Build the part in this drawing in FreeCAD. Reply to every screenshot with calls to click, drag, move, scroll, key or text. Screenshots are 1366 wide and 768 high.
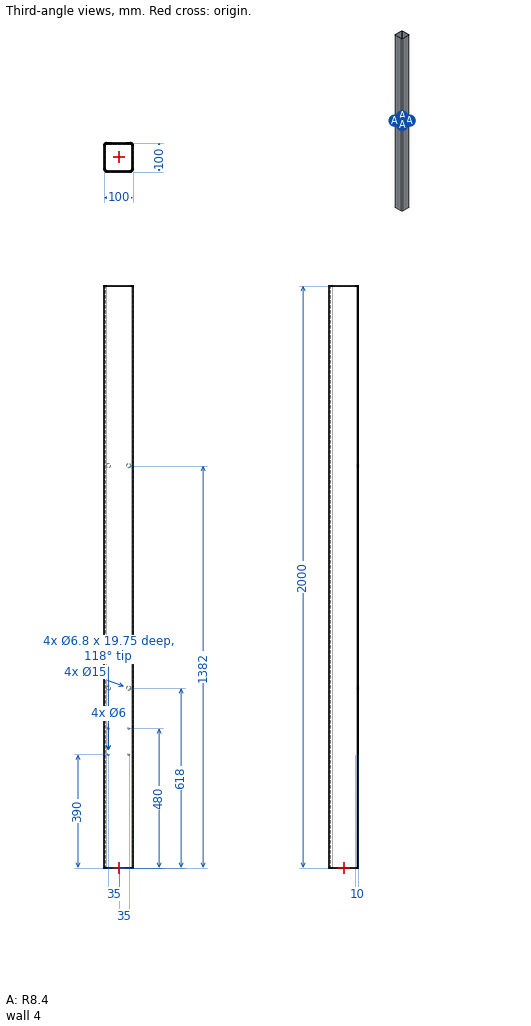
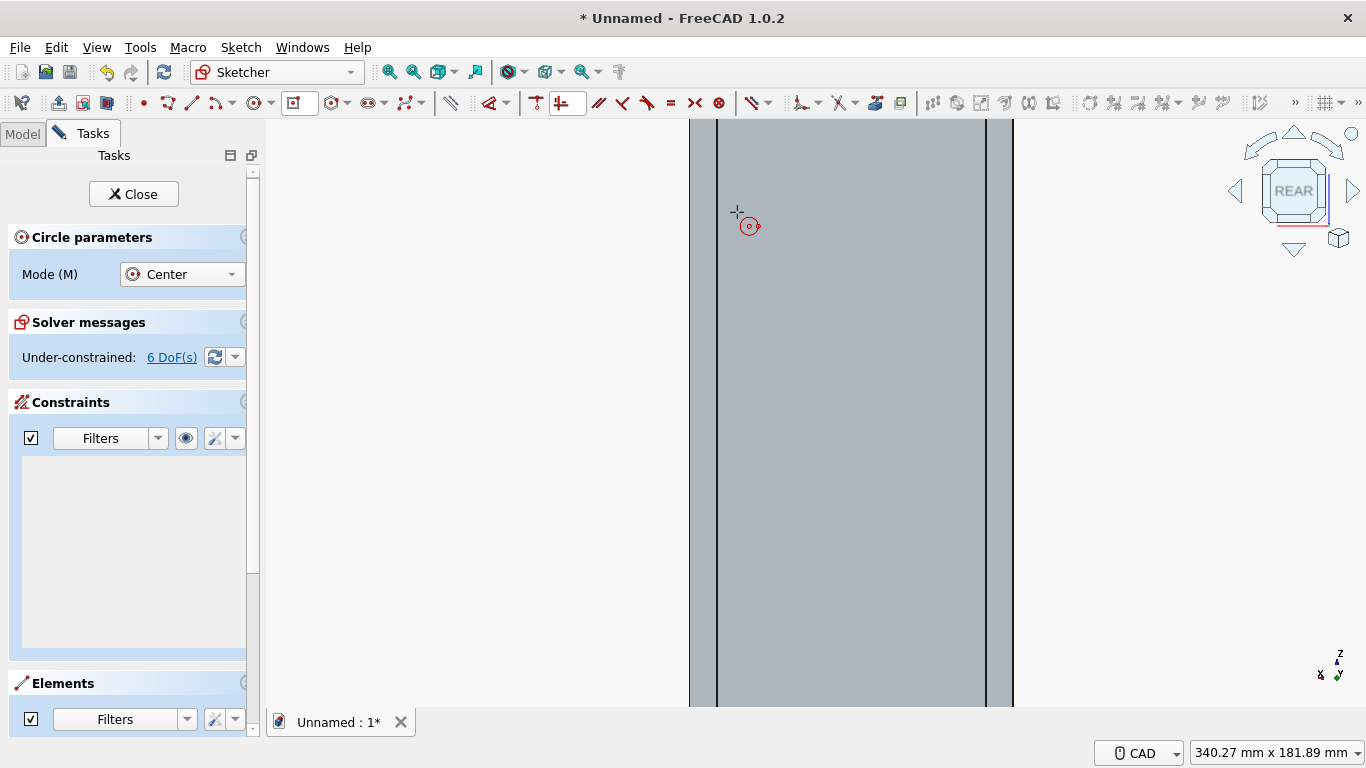
scroll(737, 212, down, 12)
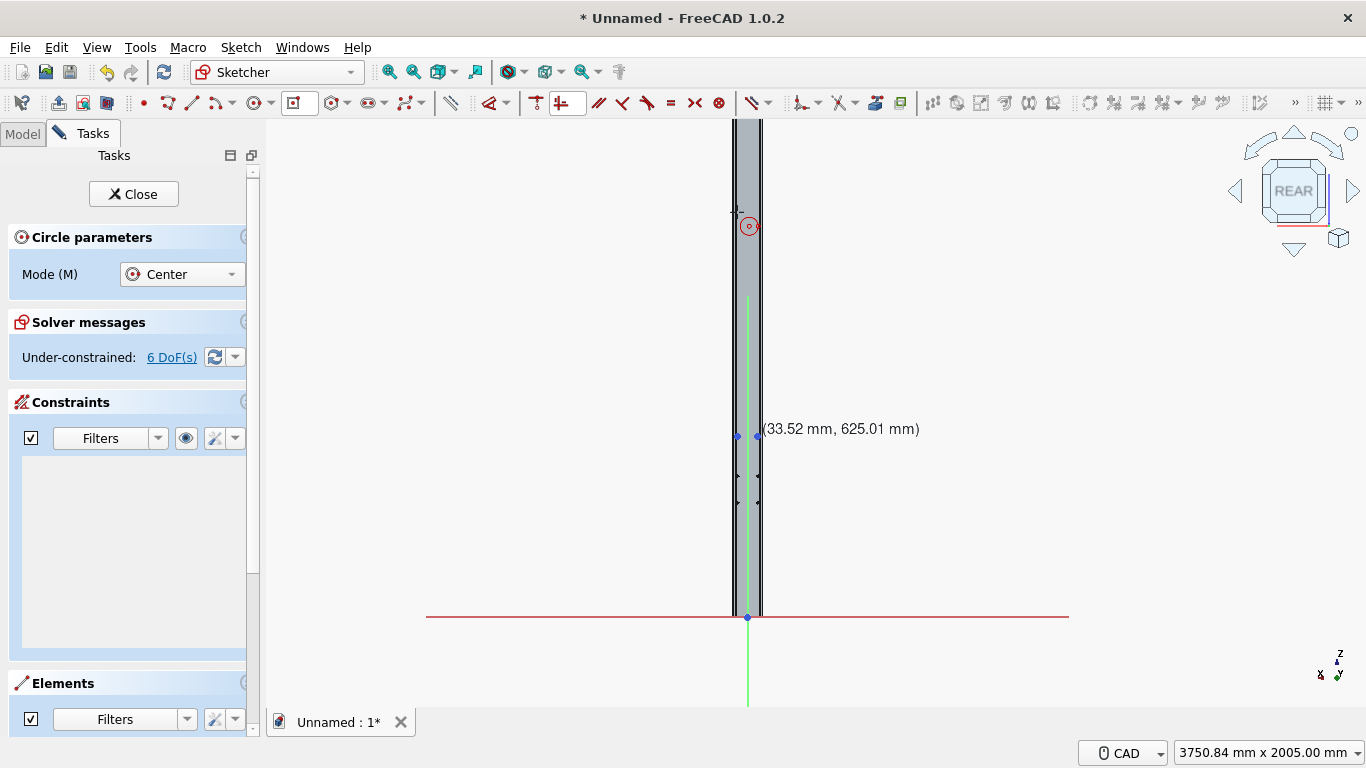
scroll(737, 212, up, 3)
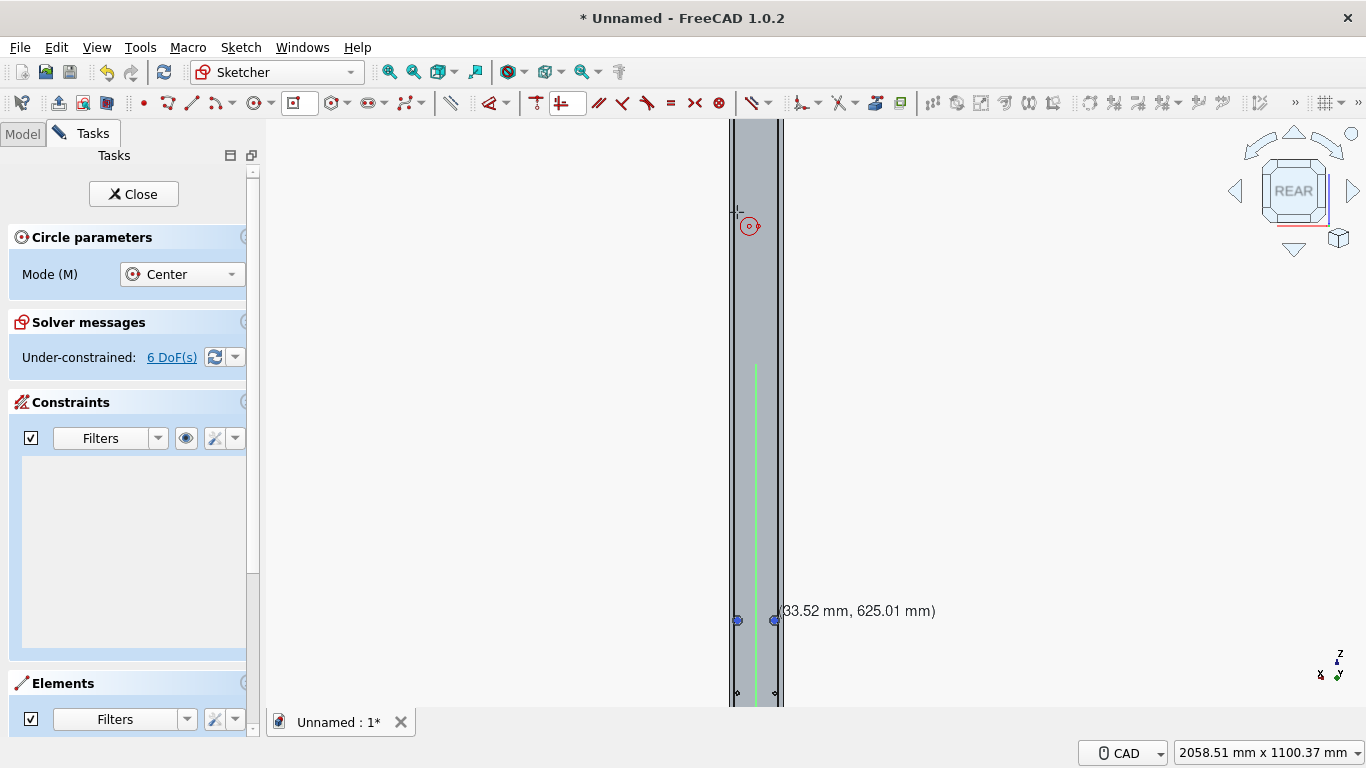
click(738, 211)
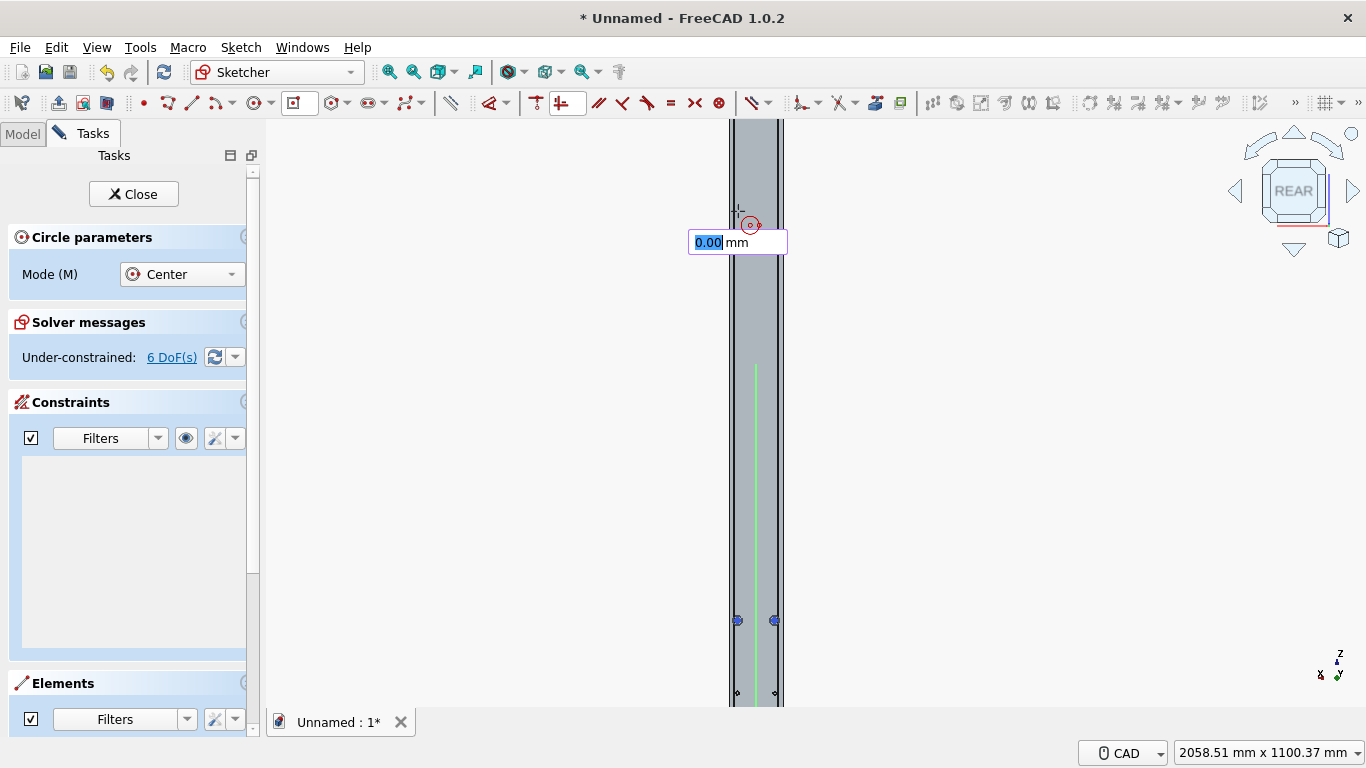
scroll(740, 209, up, 7)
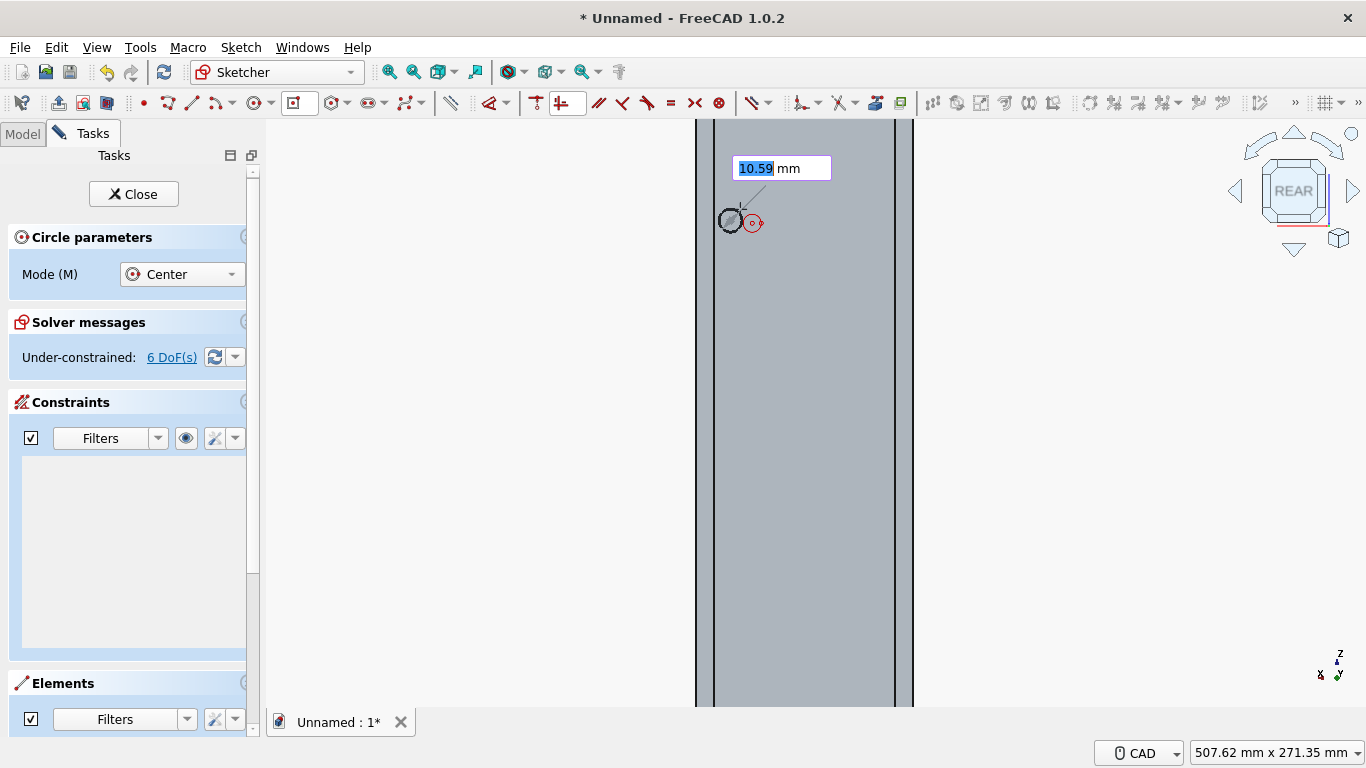
click(740, 207)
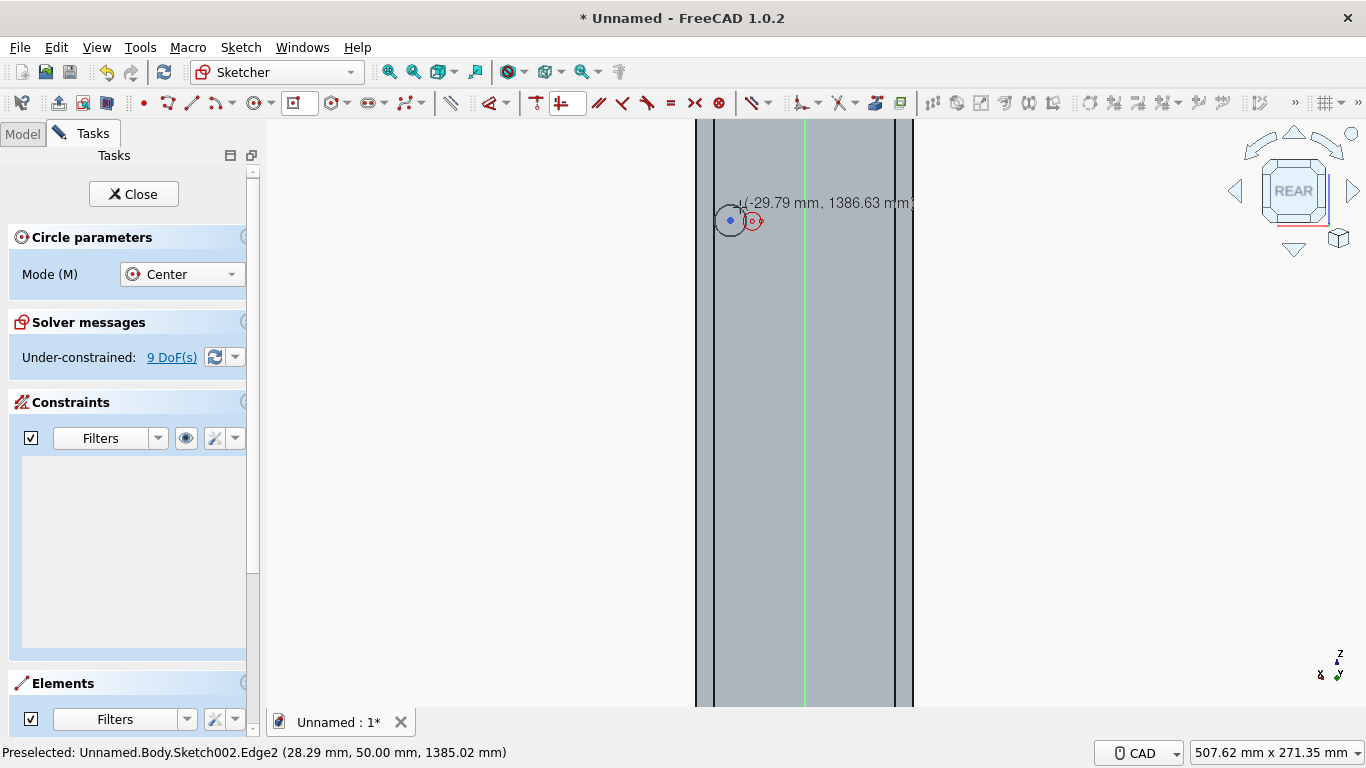
scroll(880, 218, up, 2)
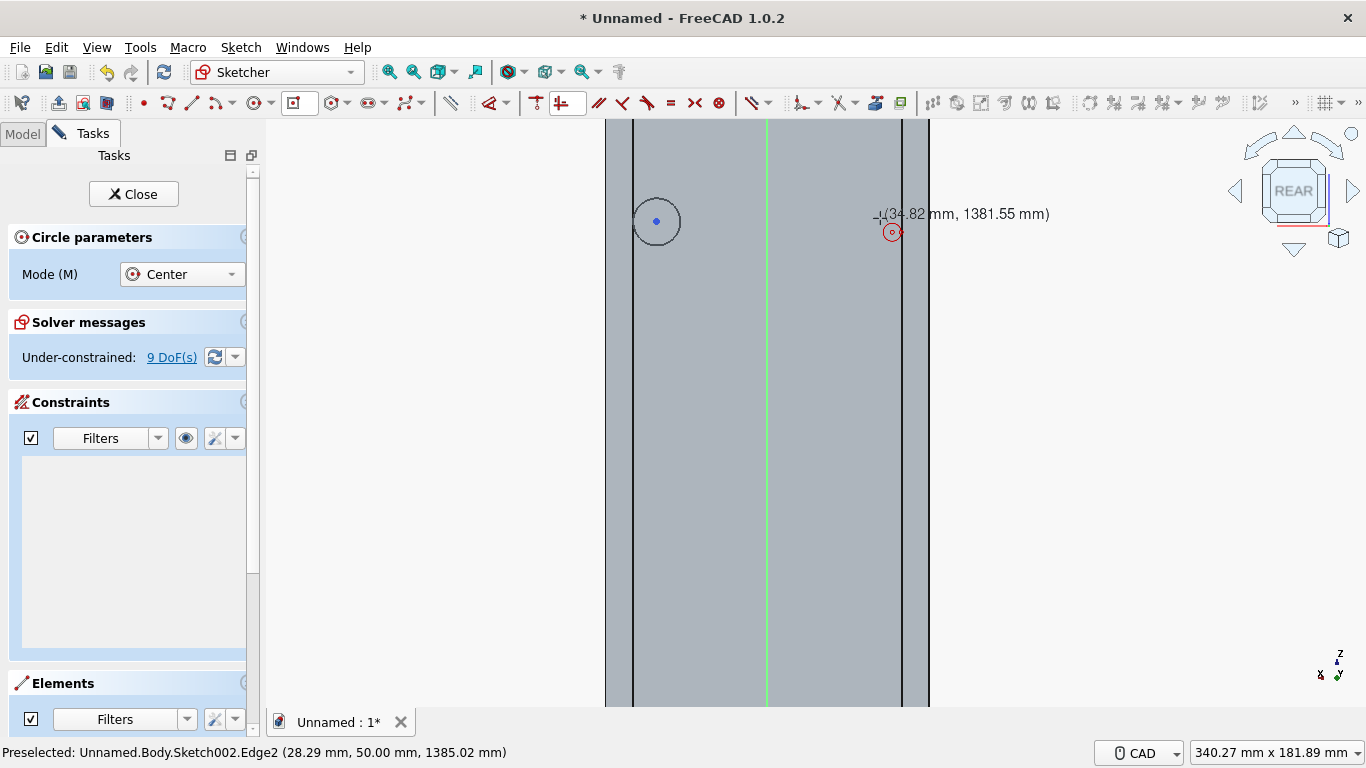
scroll(746, 211, down, 12)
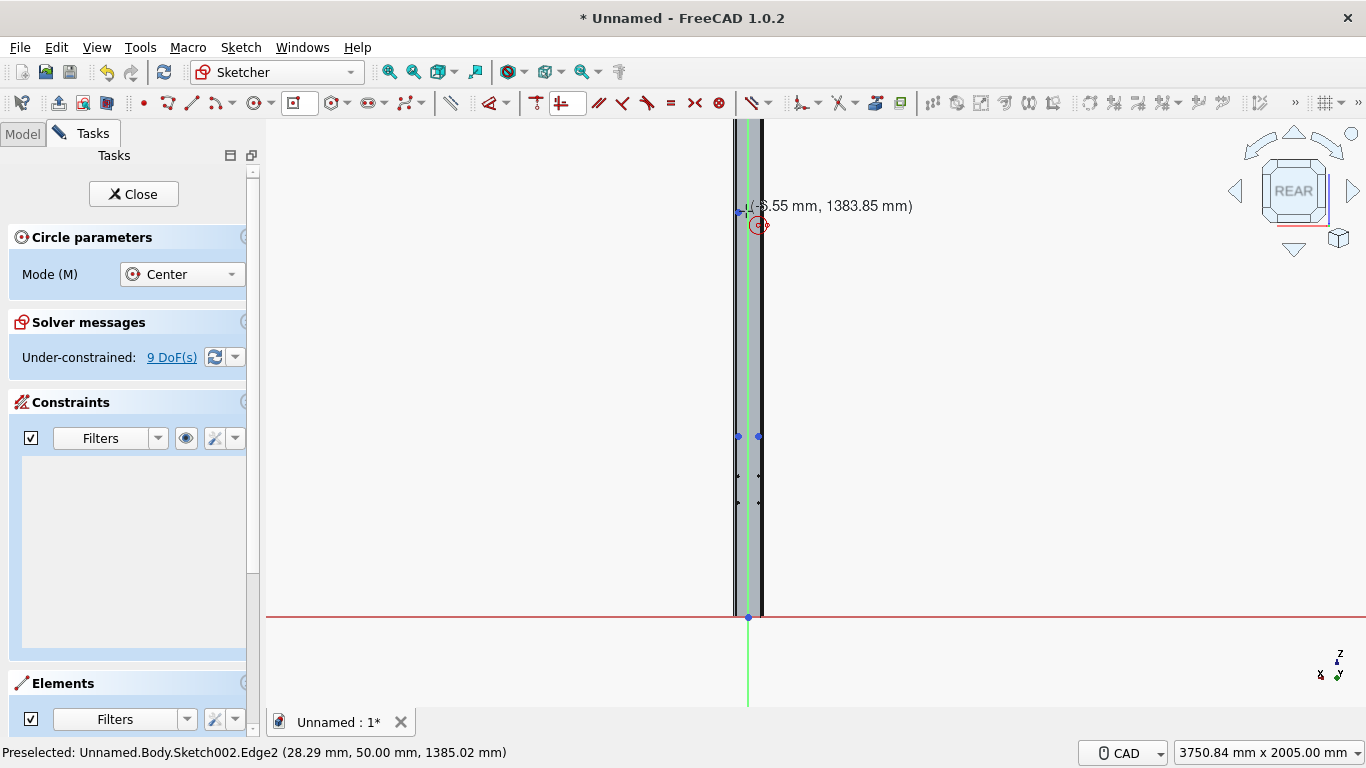
scroll(759, 212, up, 3)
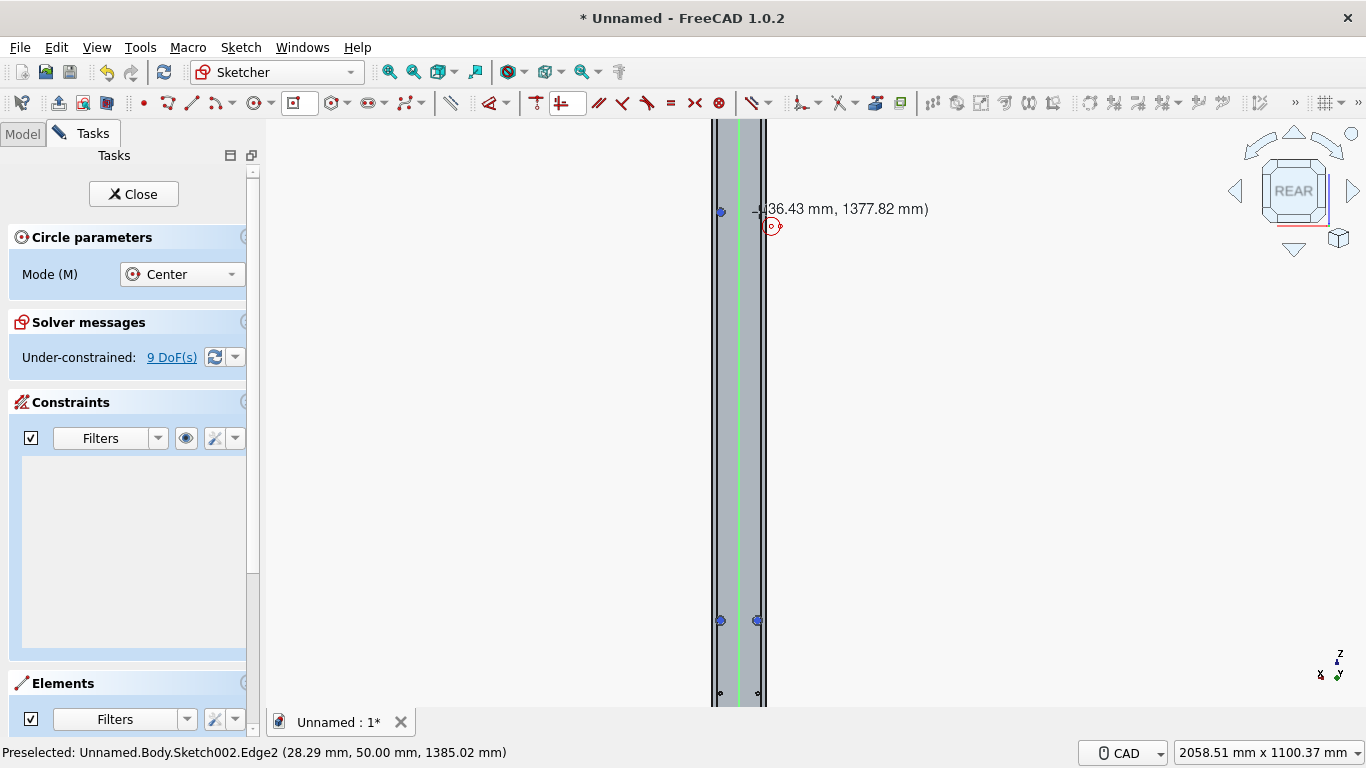
click(758, 211)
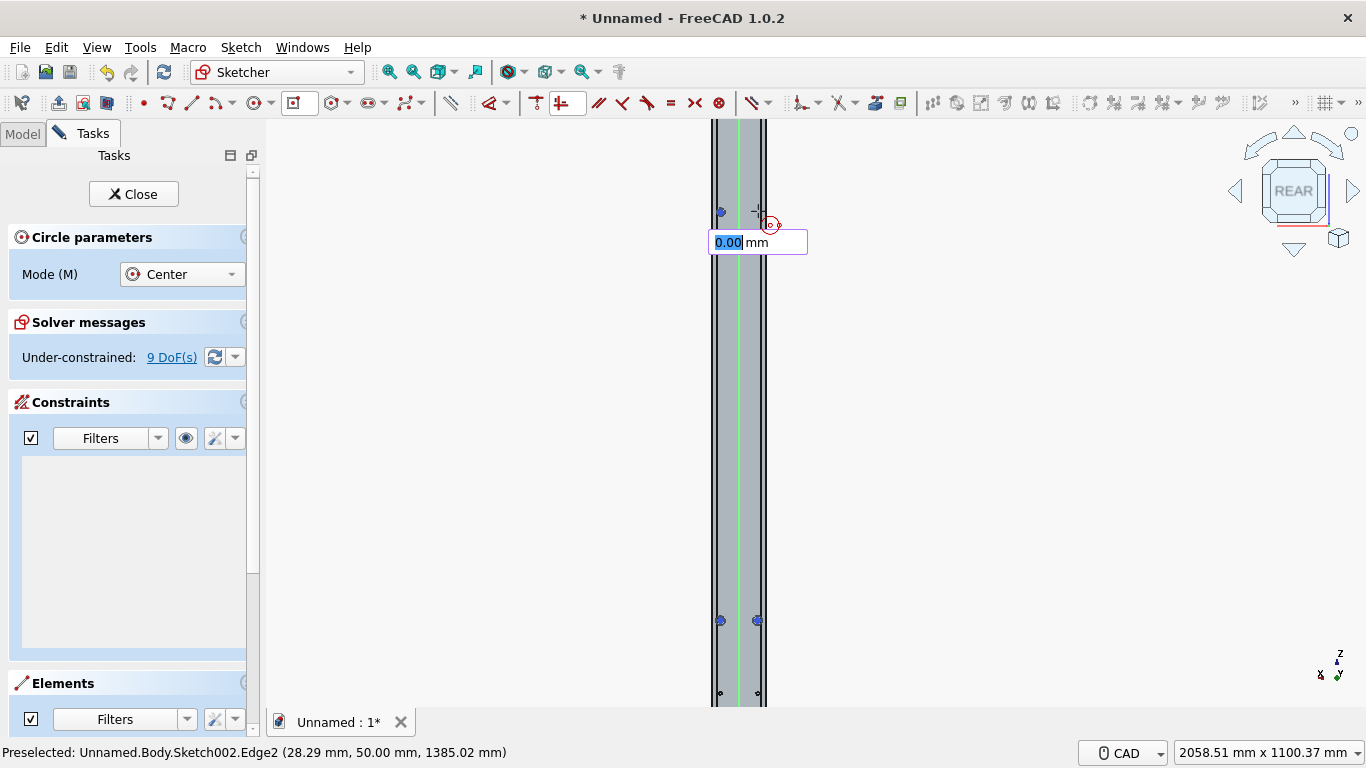
scroll(761, 209, up, 7)